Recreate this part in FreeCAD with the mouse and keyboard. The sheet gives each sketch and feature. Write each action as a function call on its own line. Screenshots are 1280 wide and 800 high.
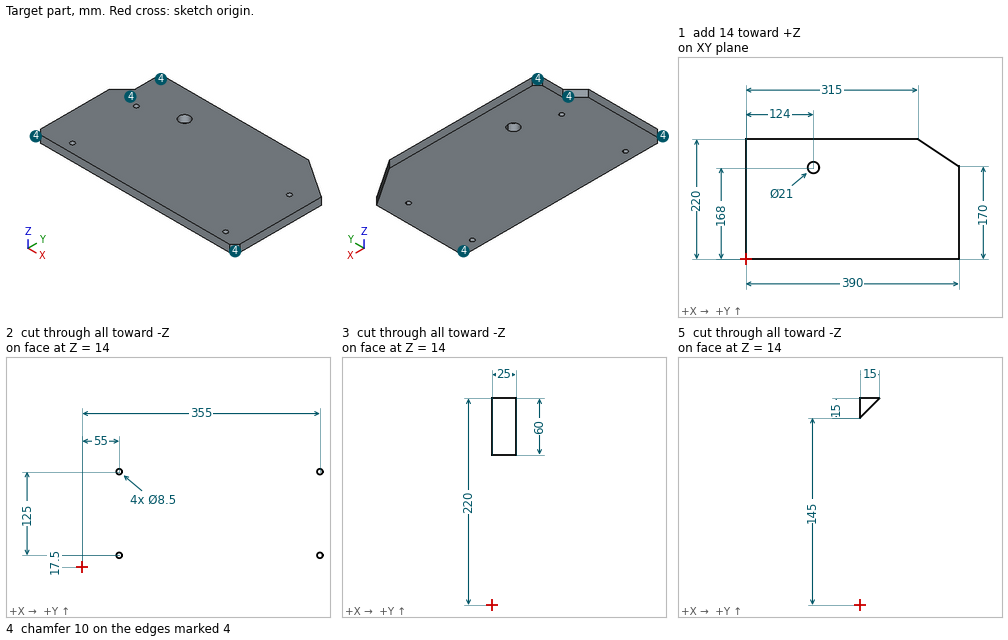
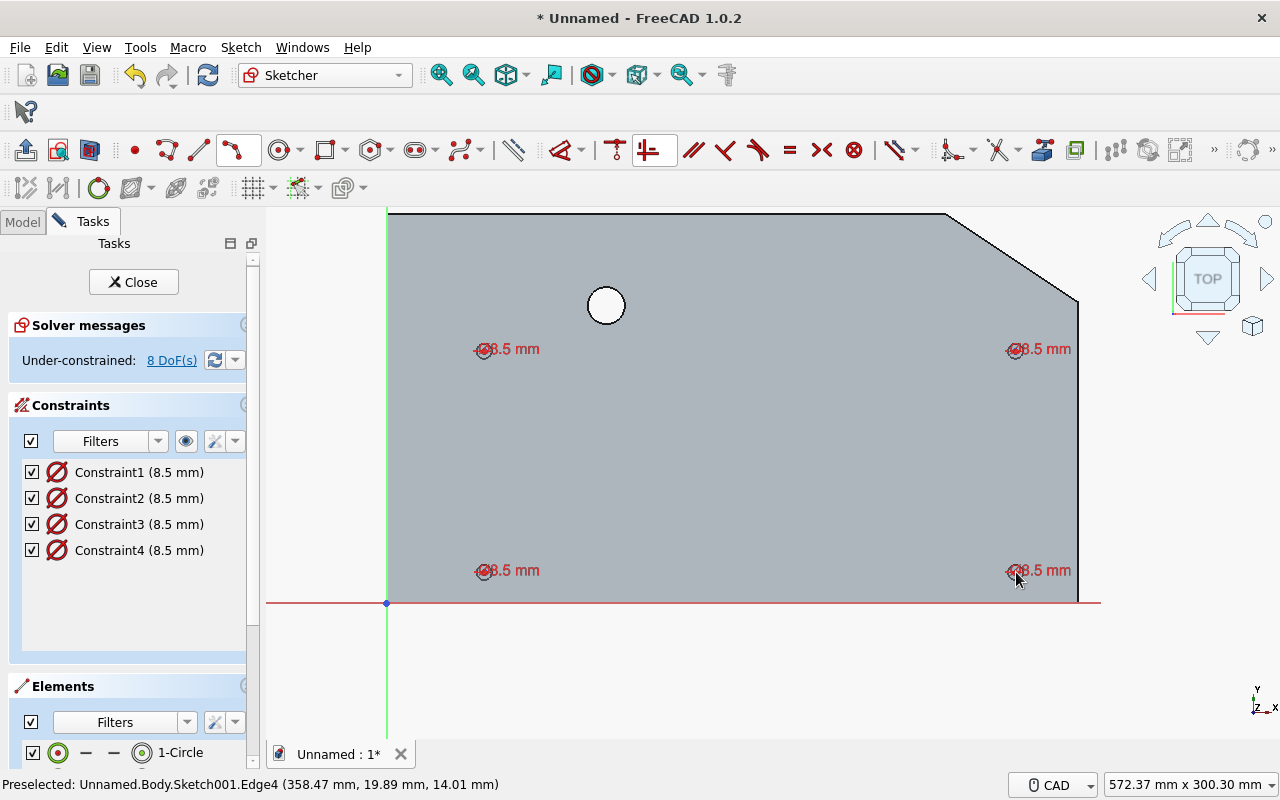
click(484, 351)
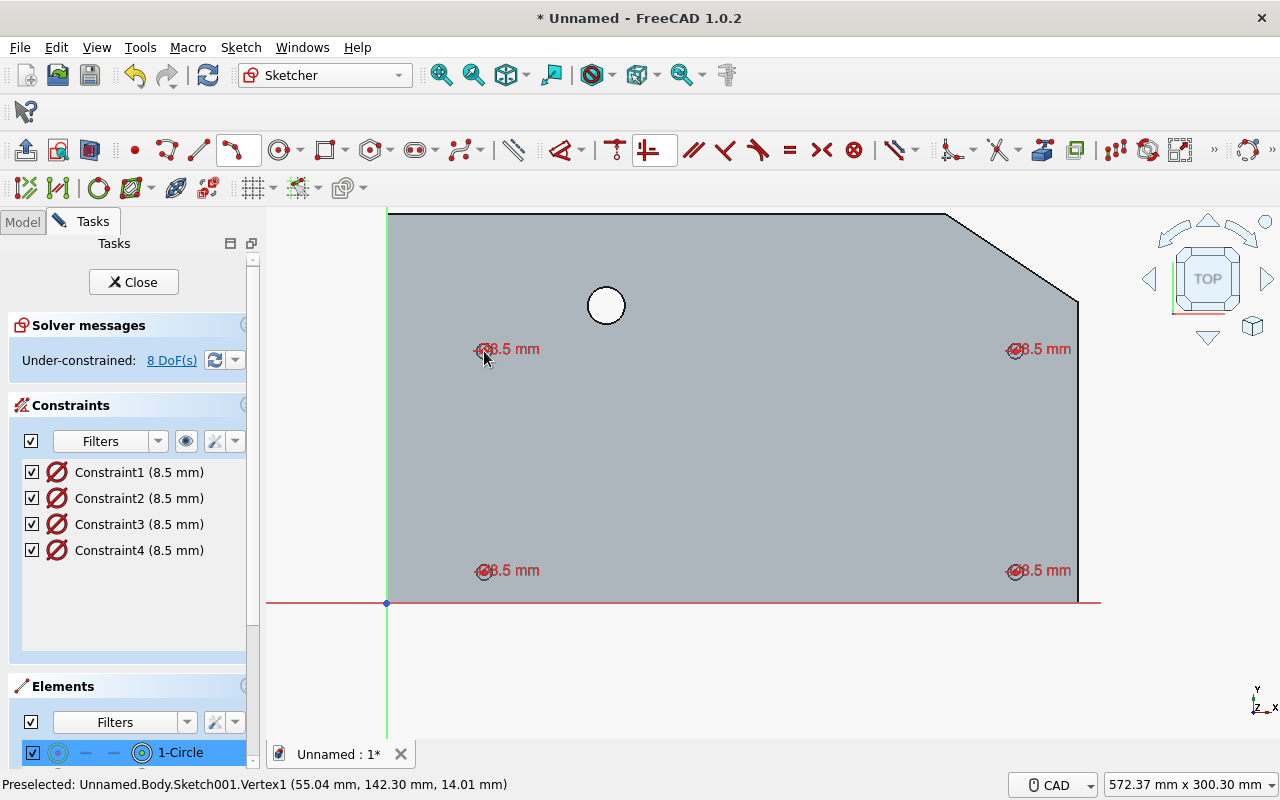
click(484, 572)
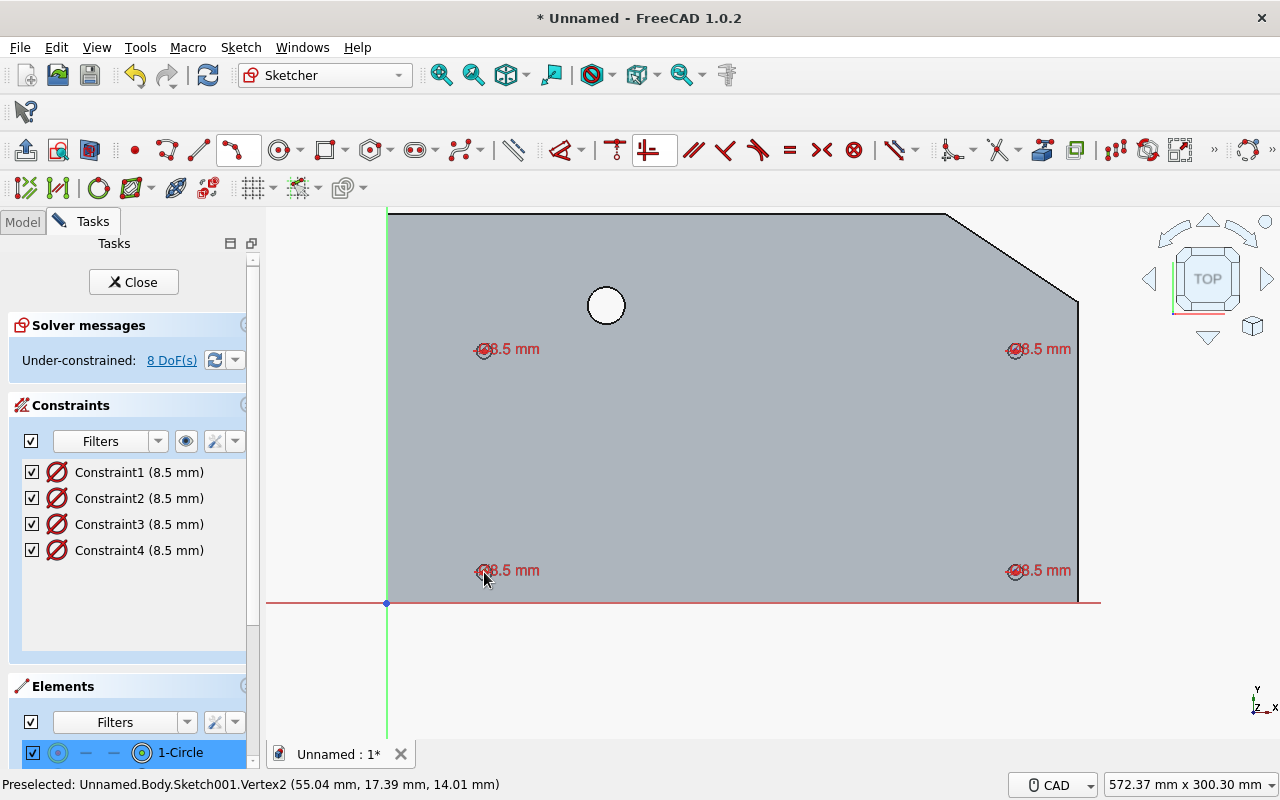
key(v)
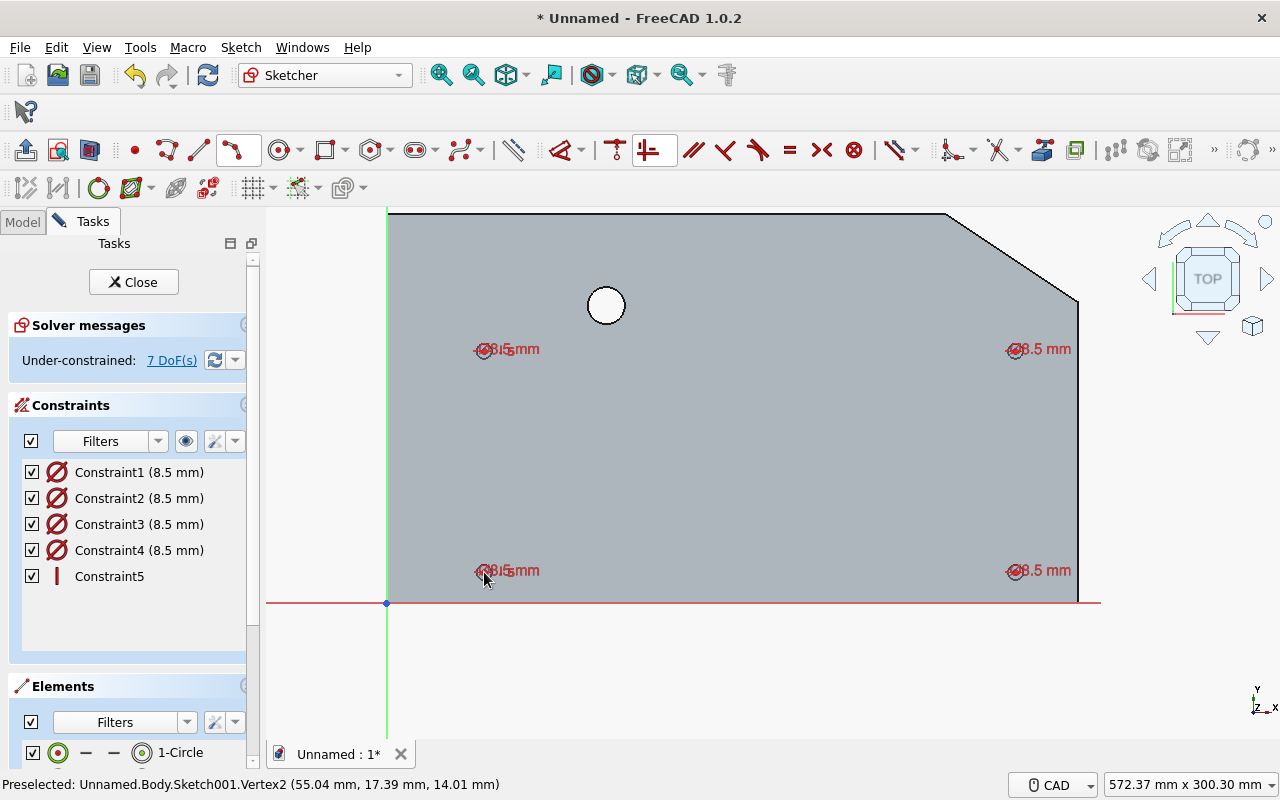
click(484, 351)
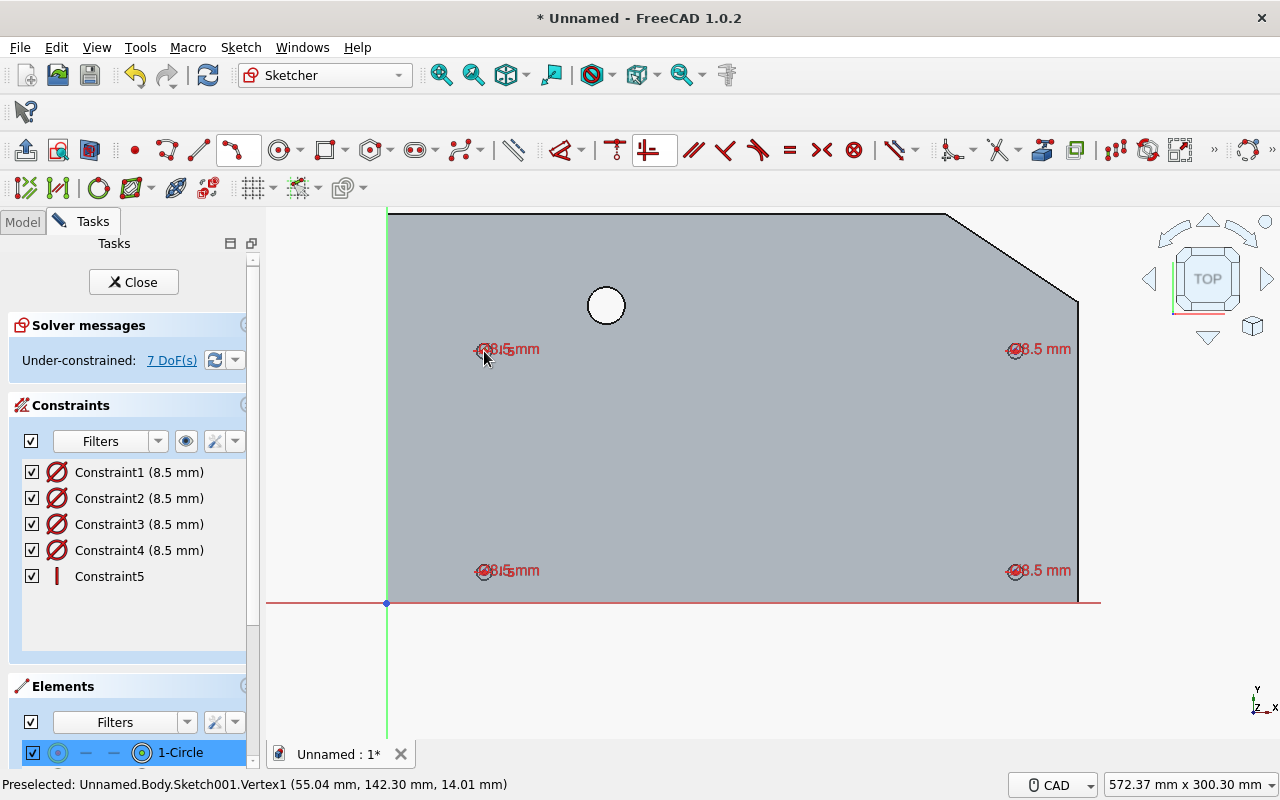
click(1016, 351)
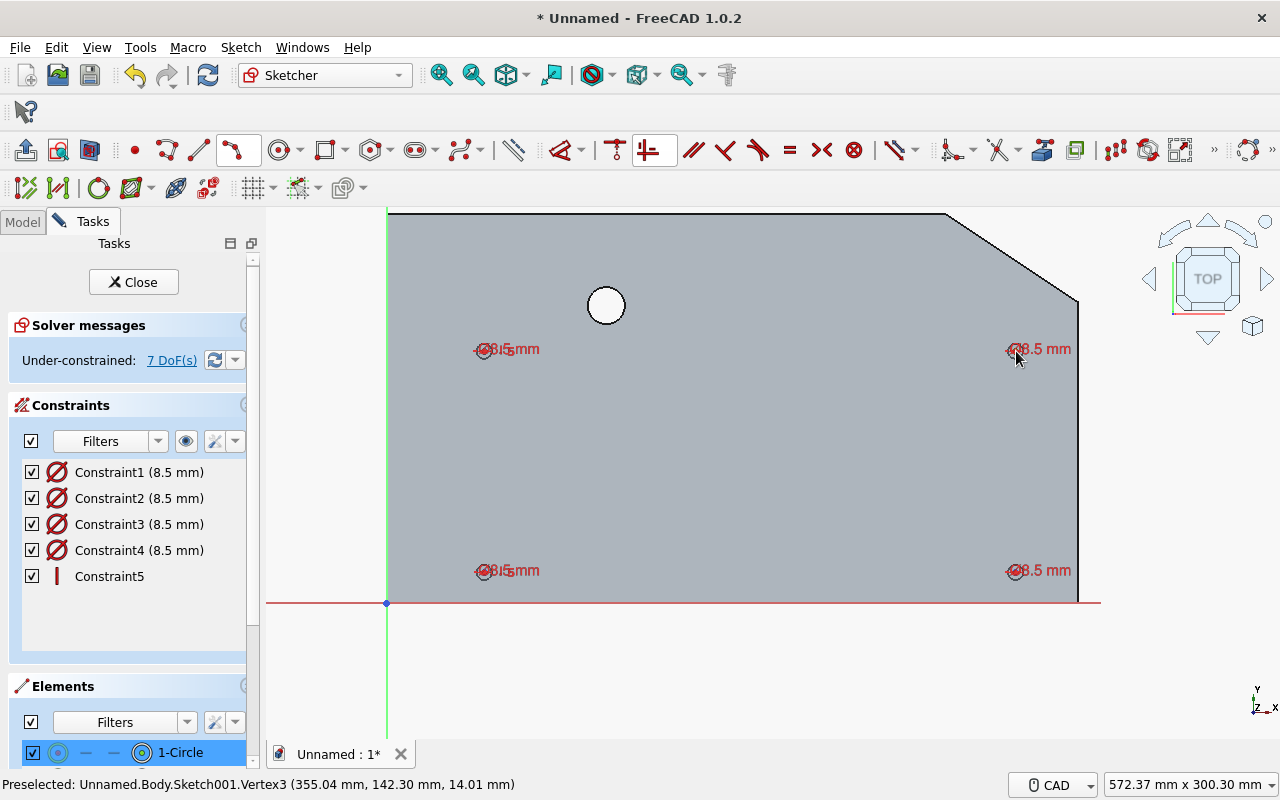
key(h)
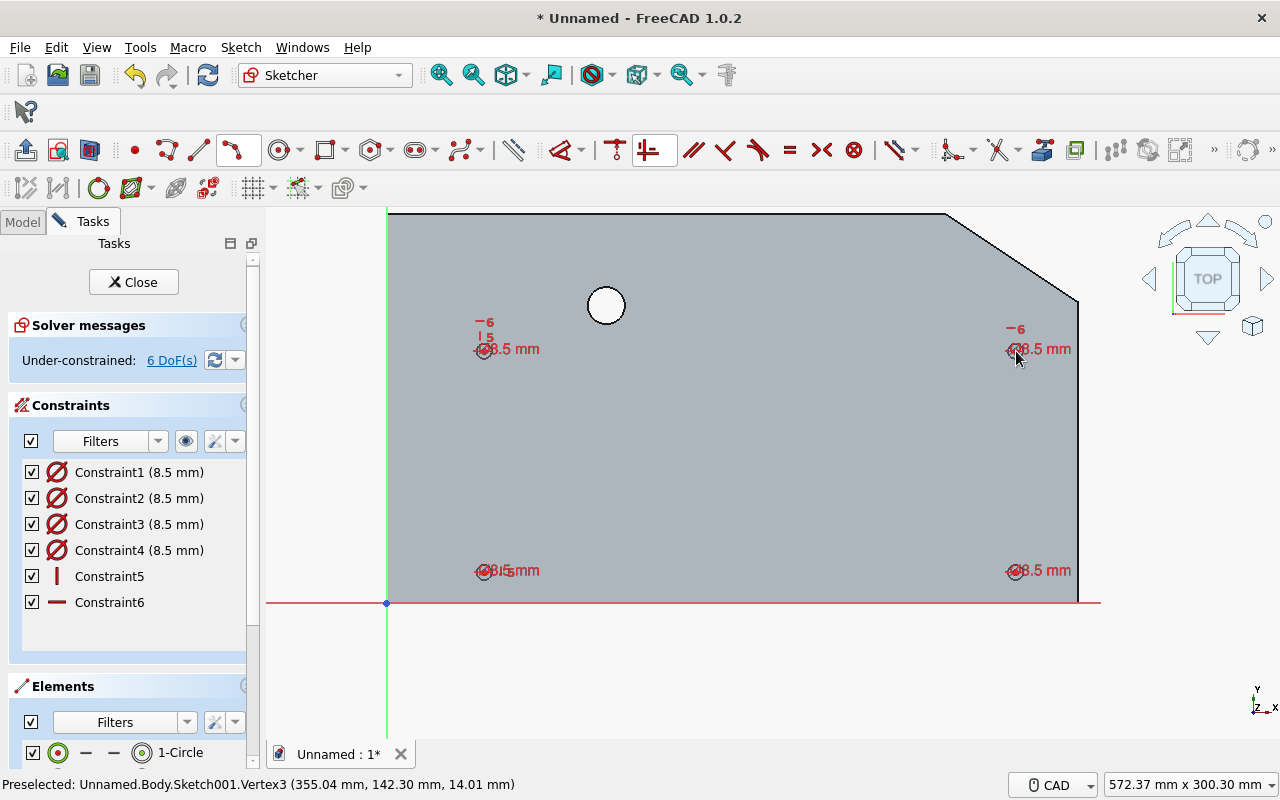
click(1016, 351)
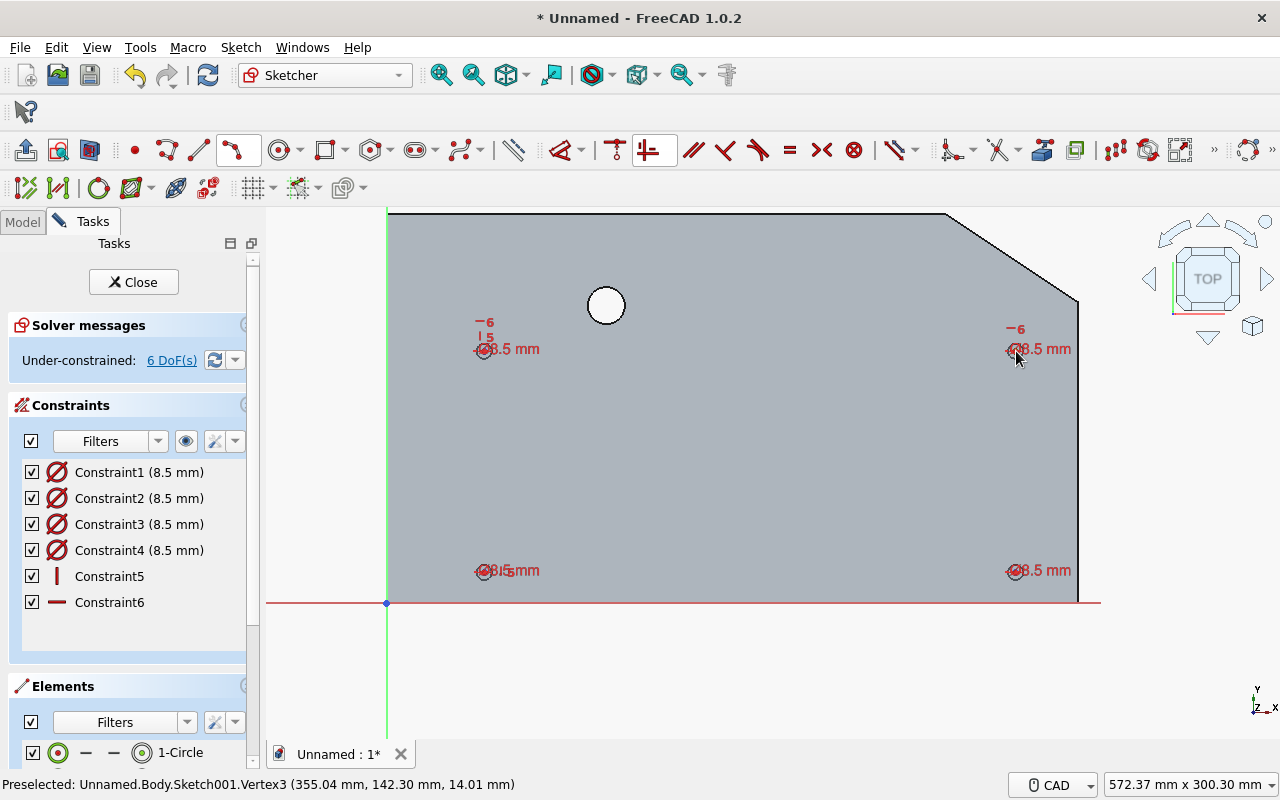
click(1016, 572)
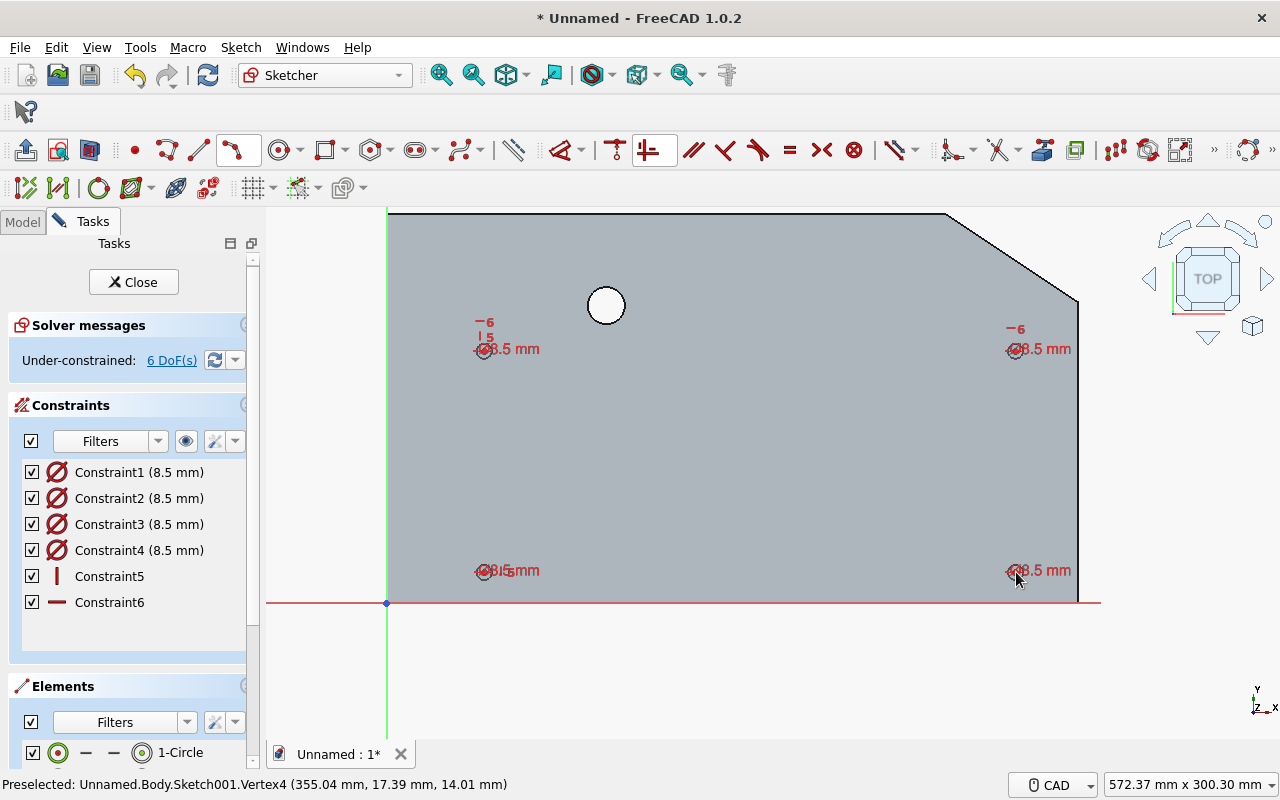
key(v)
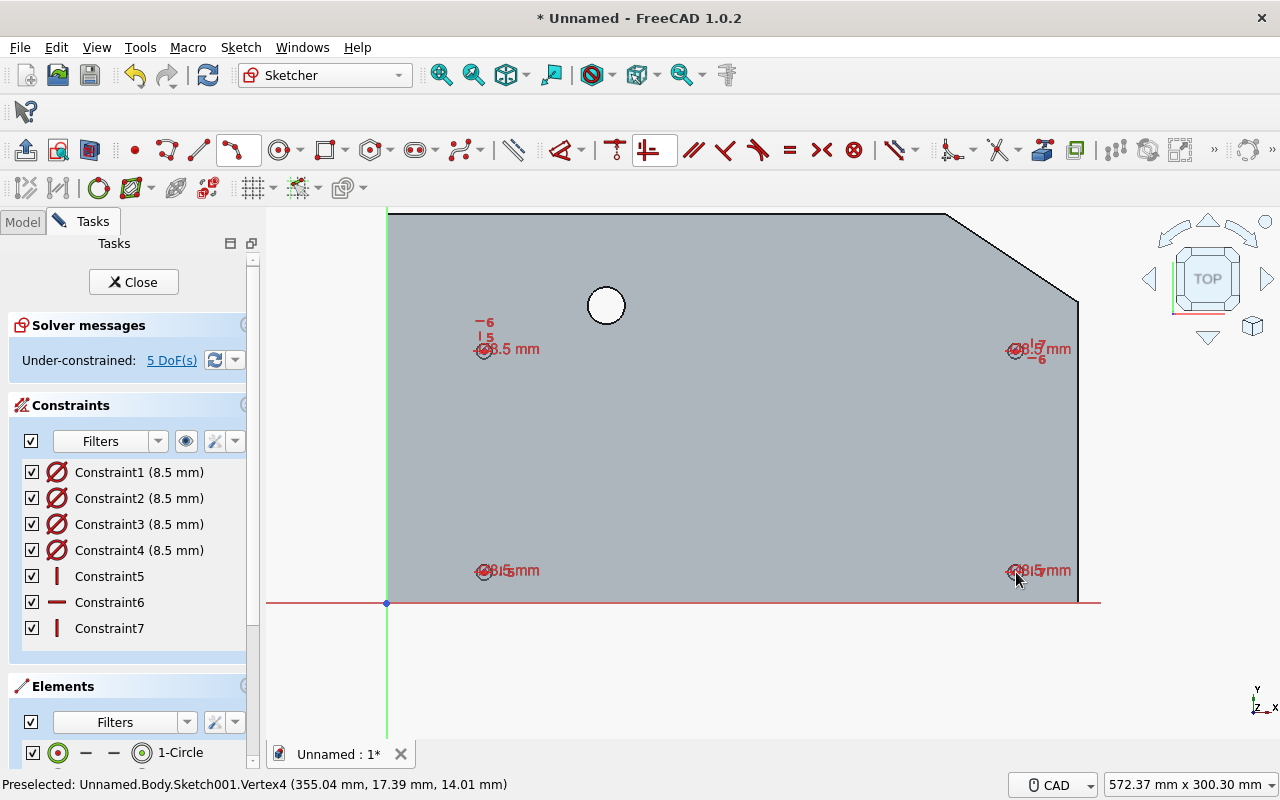
click(484, 572)